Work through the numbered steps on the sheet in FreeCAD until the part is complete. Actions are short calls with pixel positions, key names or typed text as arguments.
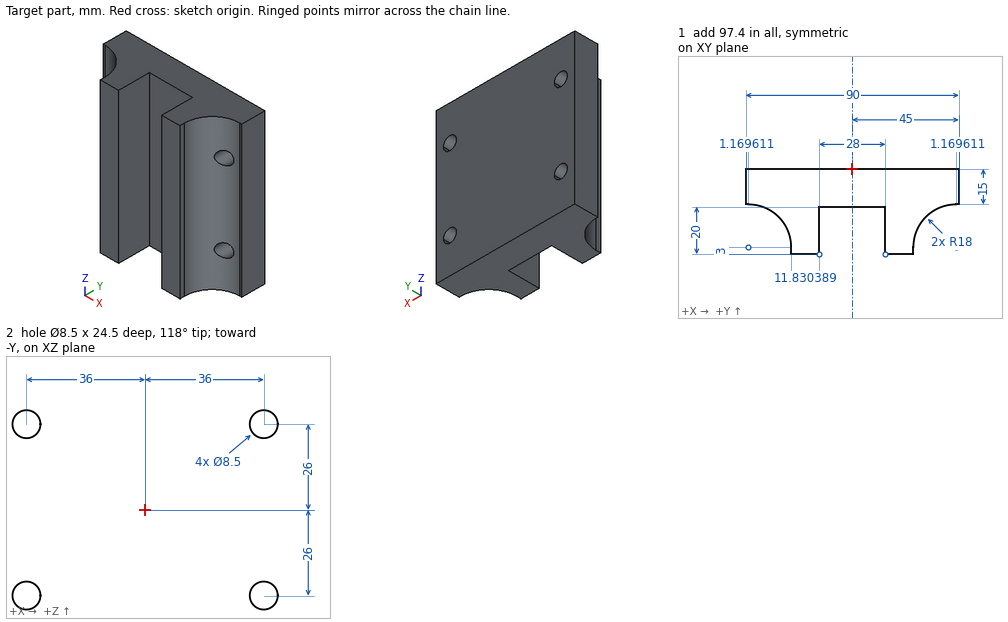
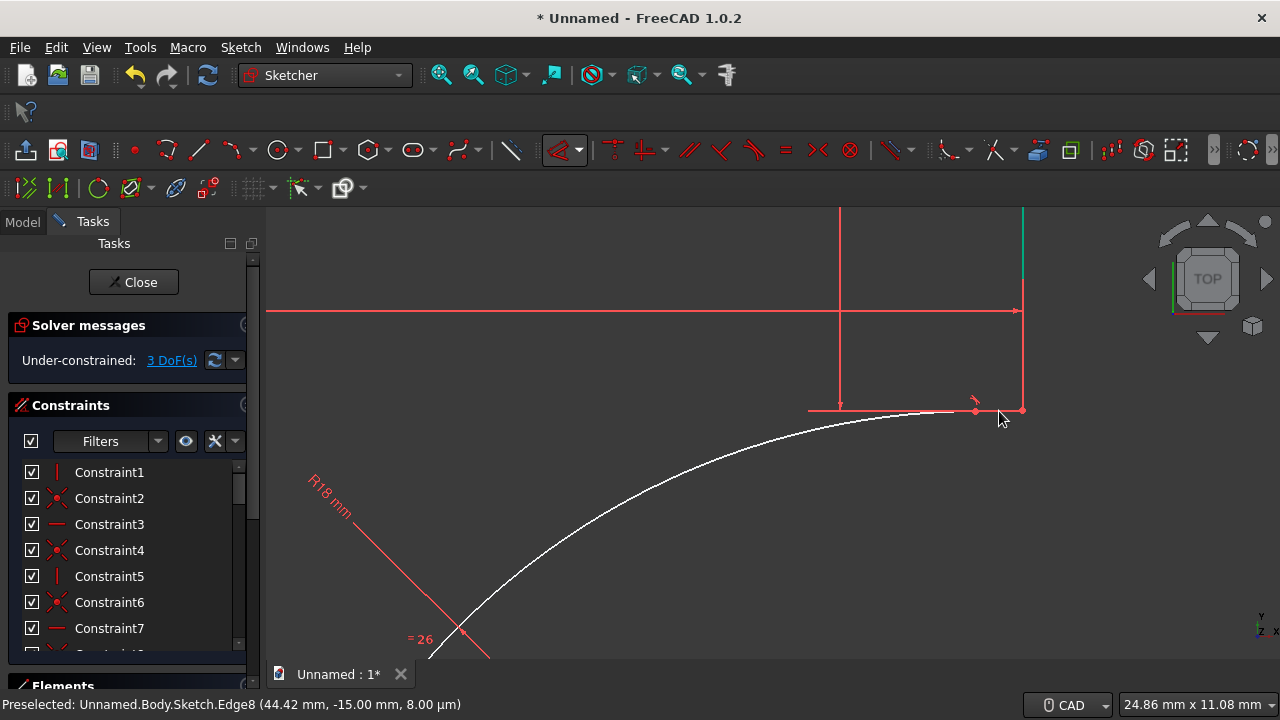
key(l)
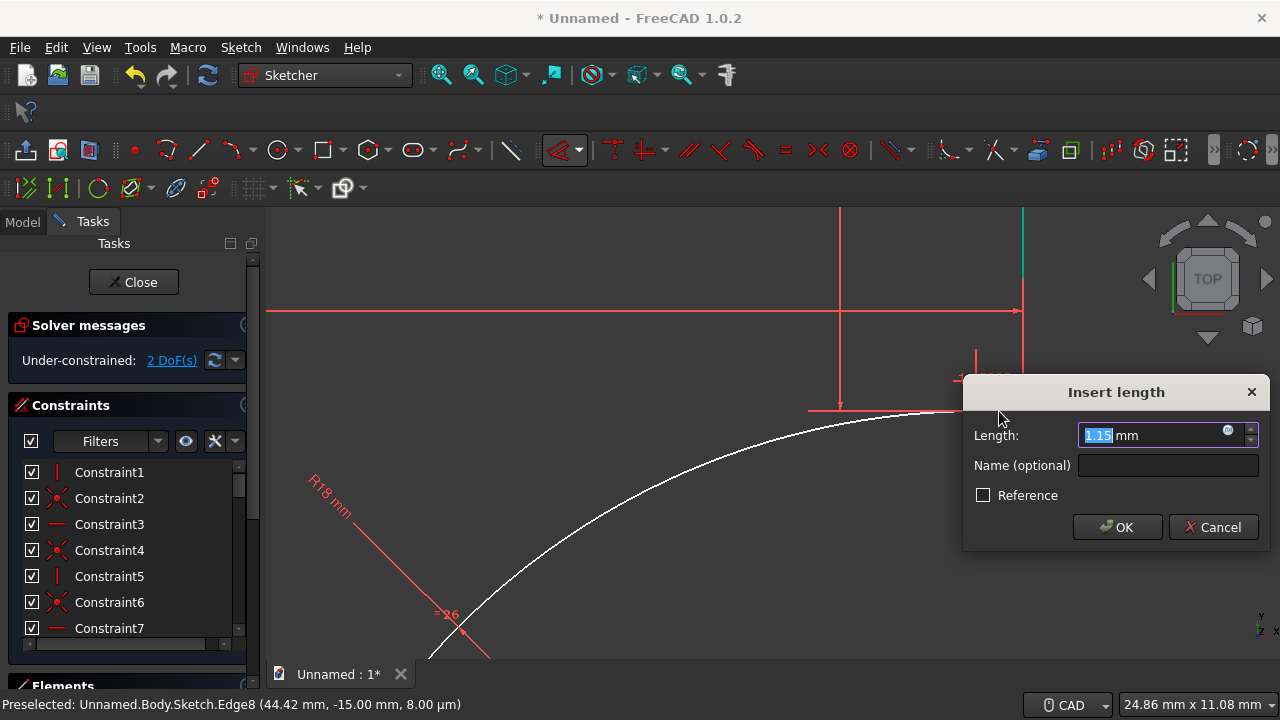
text(1.169611)
key(Return)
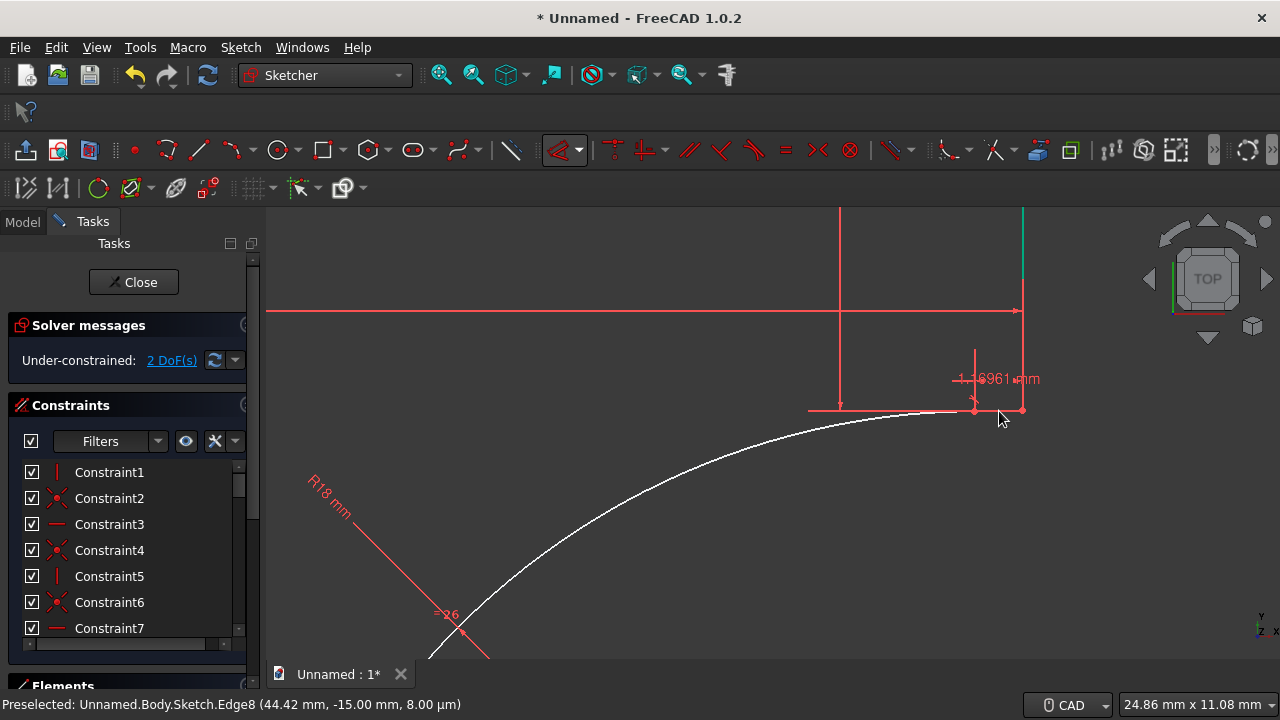
scroll(1005, 413, down, 9)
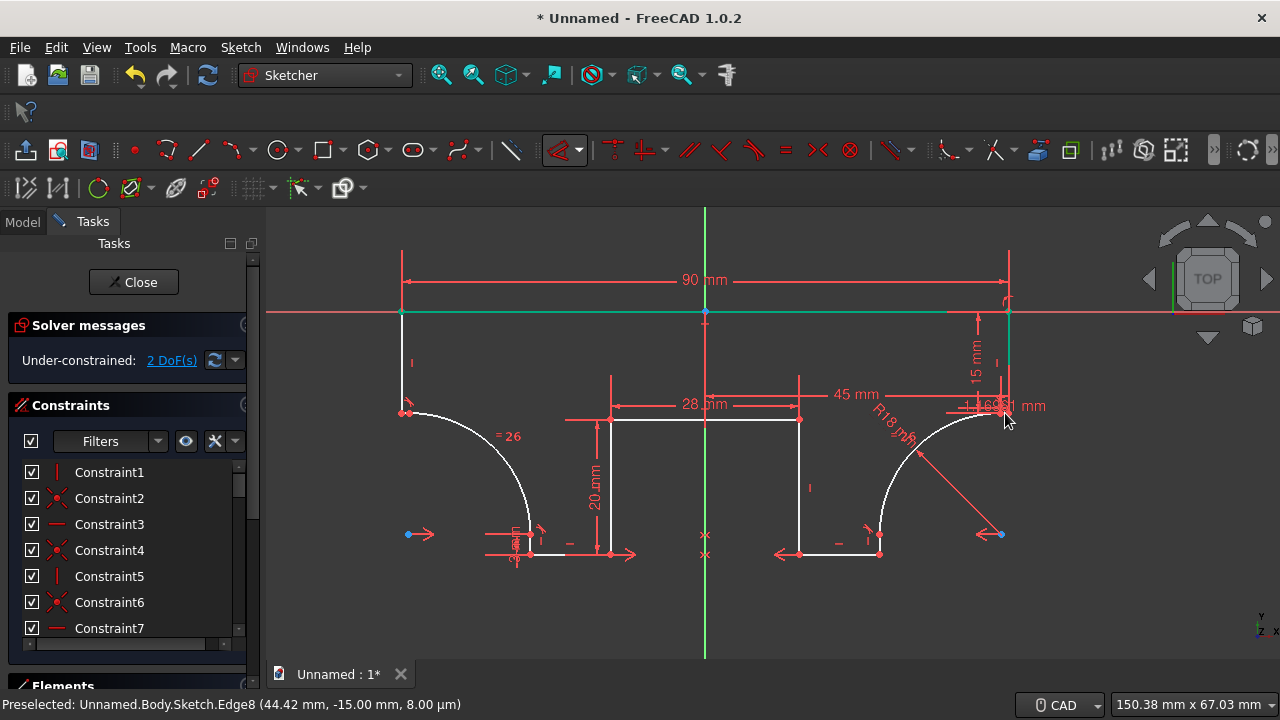
scroll(404, 413, up, 9)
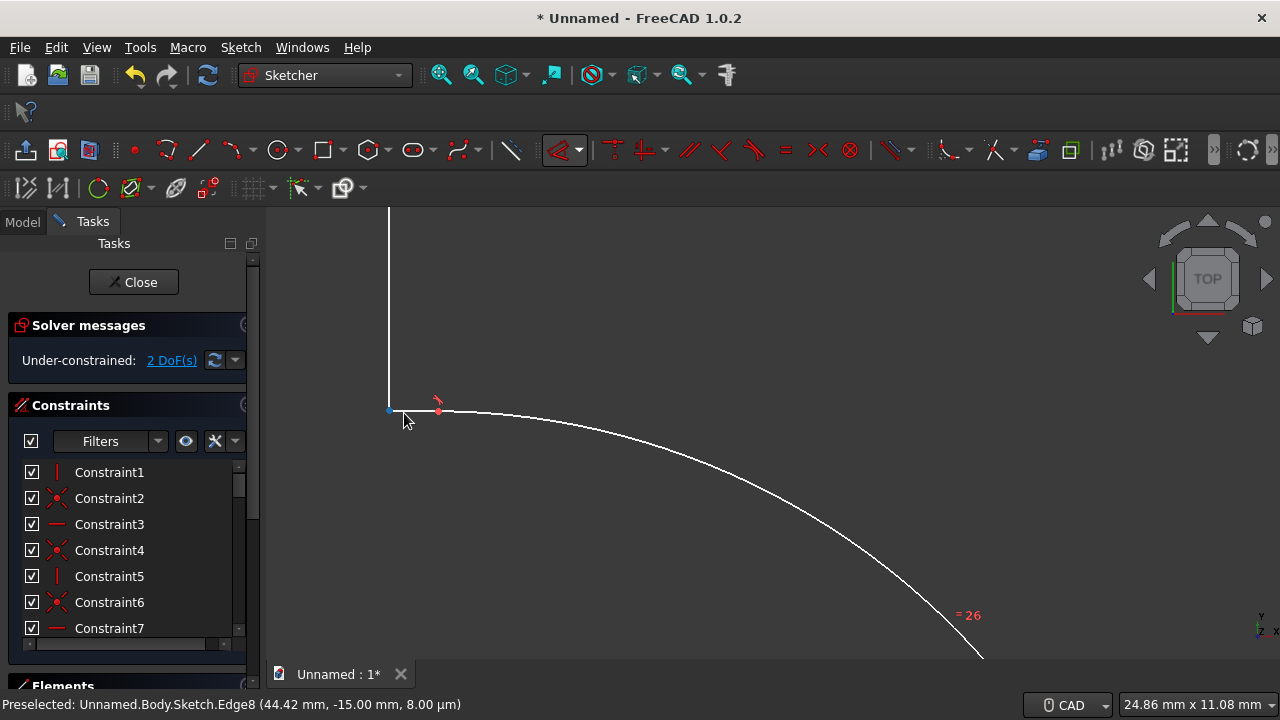
click(404, 411)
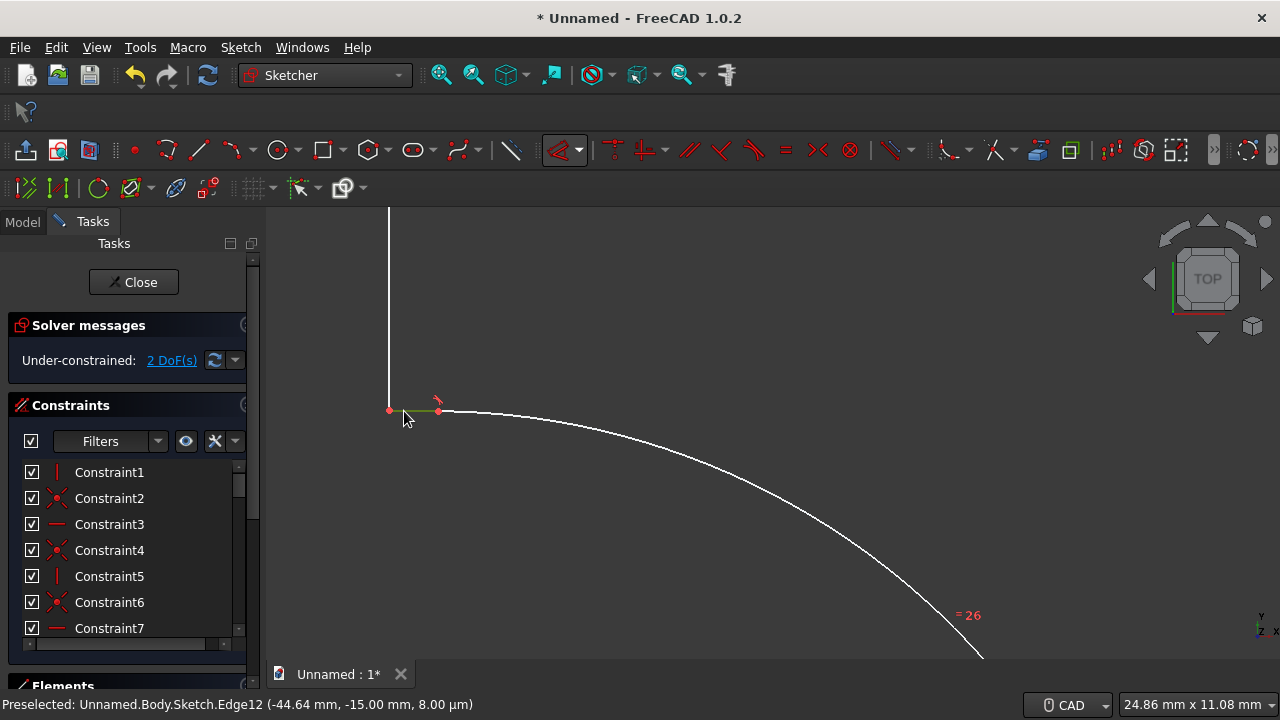
click(582, 150)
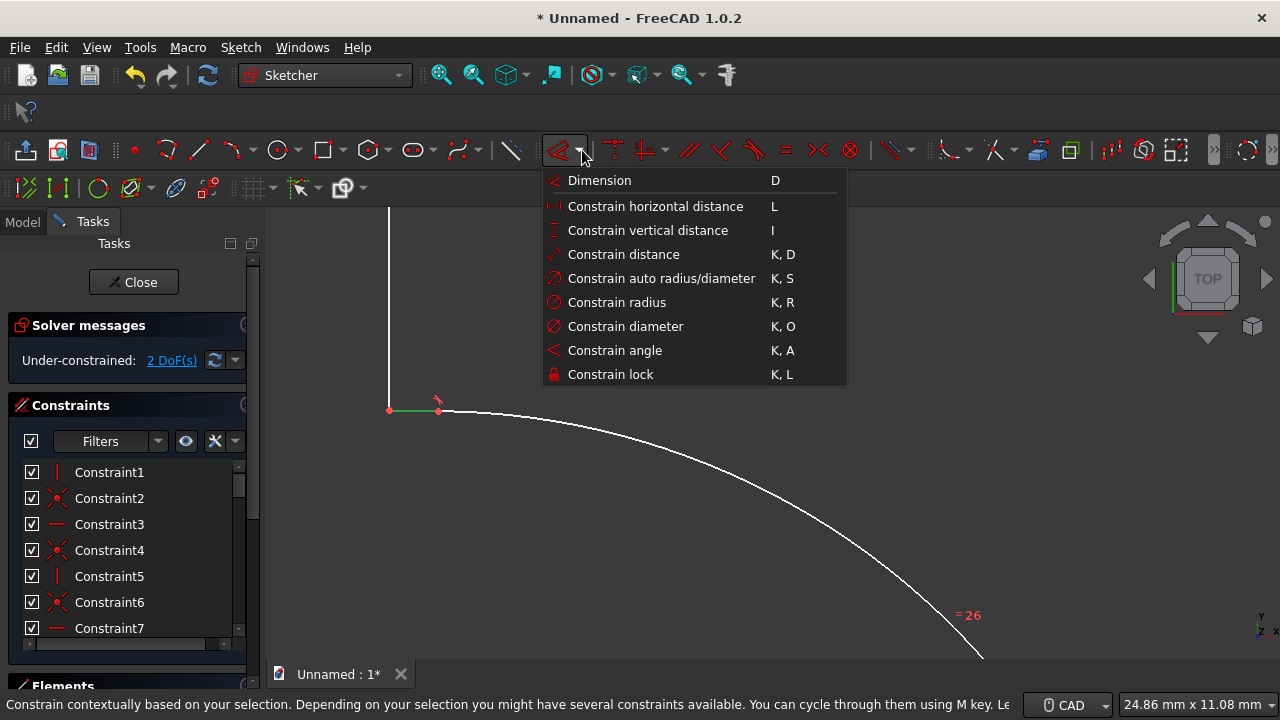
click(695, 206)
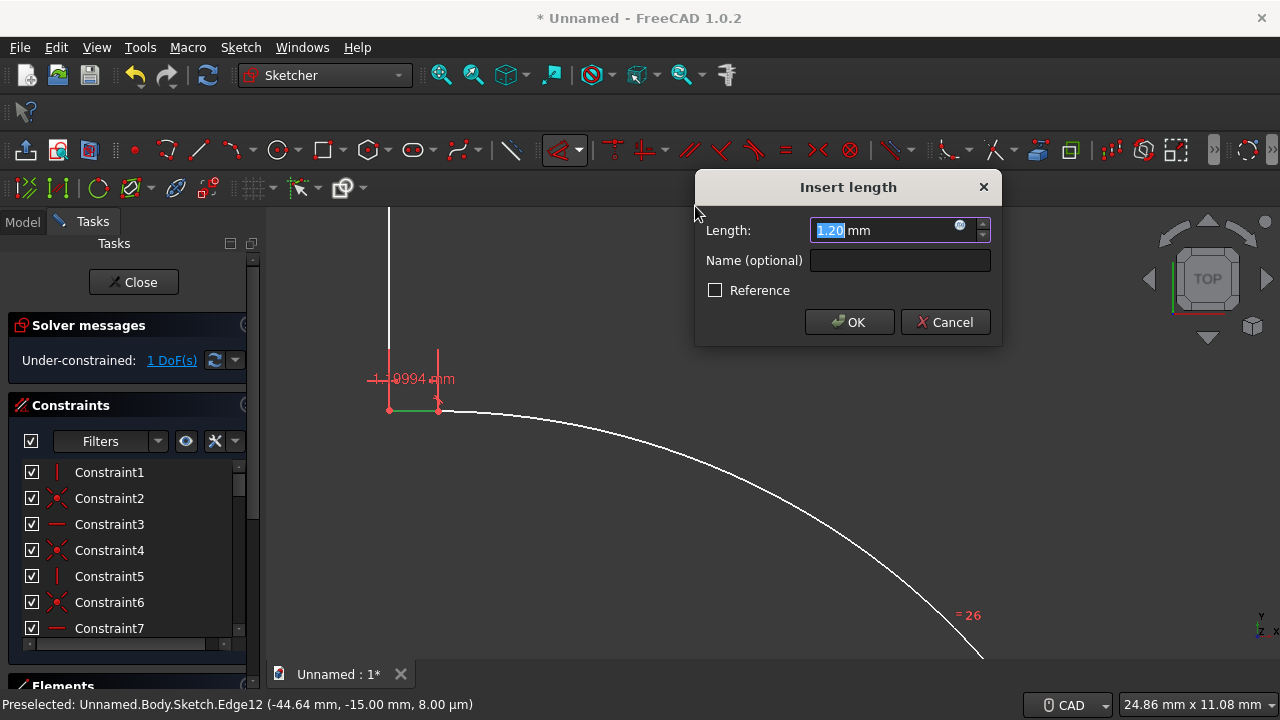
text(1.169611)
key(Return)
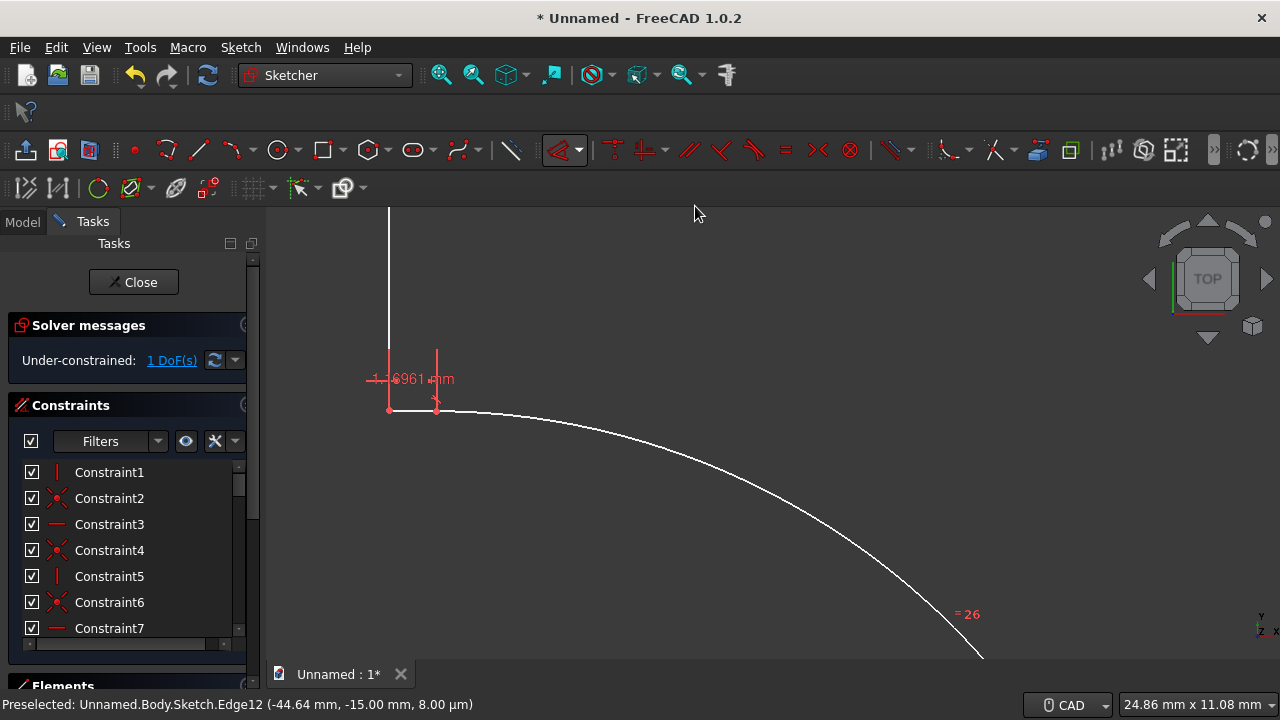
scroll(403, 413, down, 9)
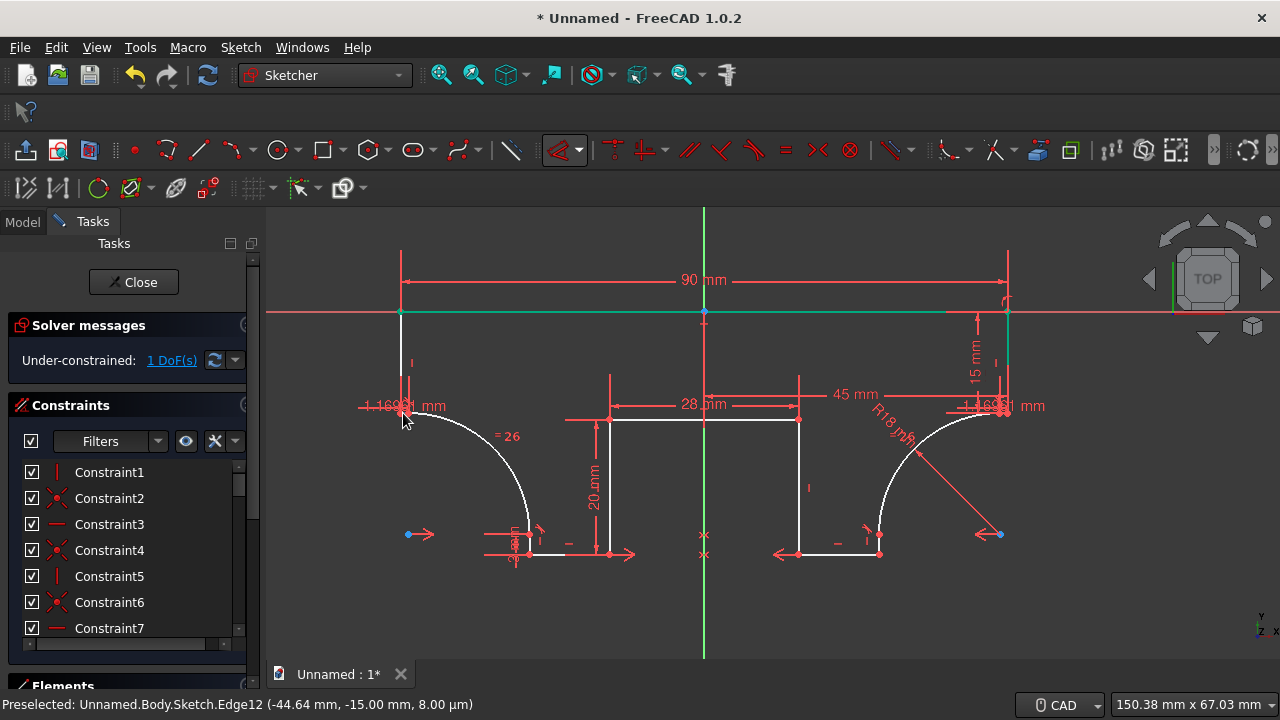
click(554, 555)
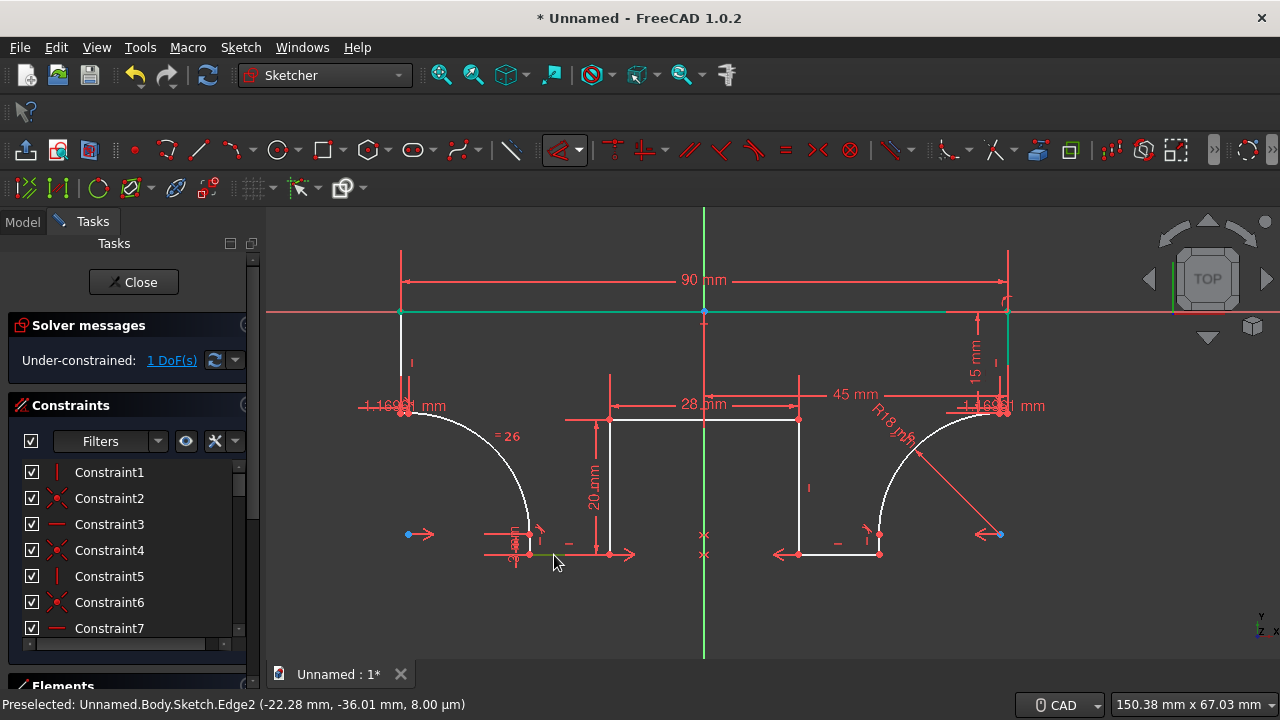
key(l)